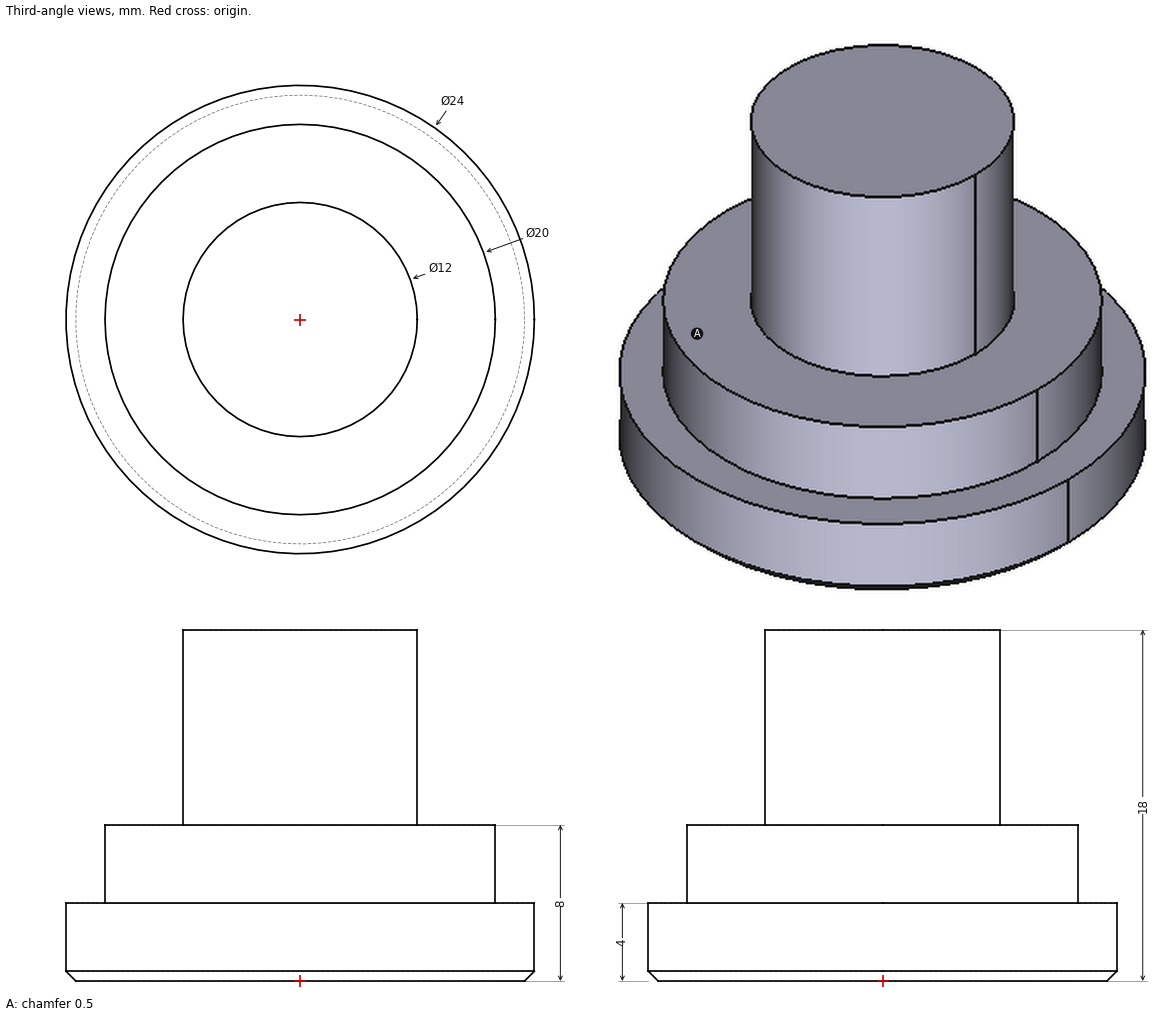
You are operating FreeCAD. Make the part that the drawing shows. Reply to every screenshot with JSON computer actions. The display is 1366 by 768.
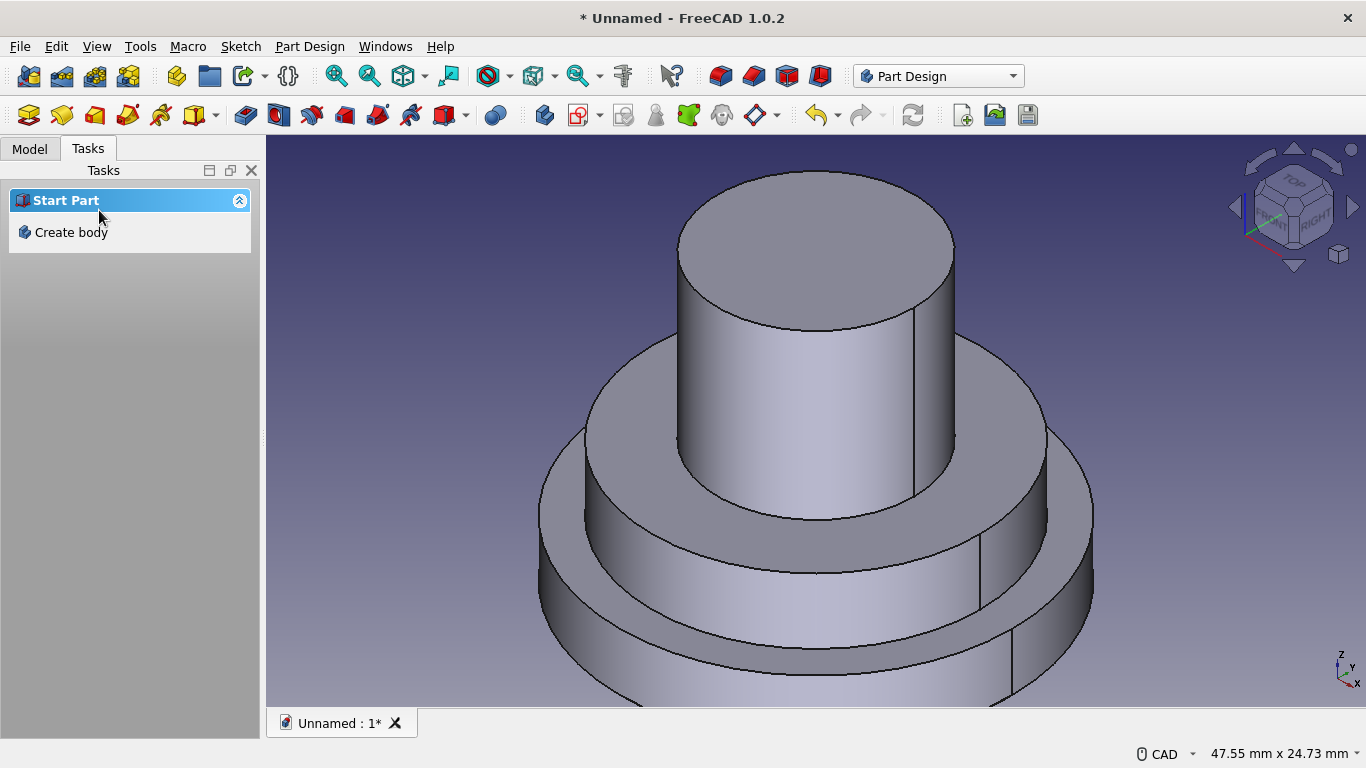
{"action": "left_click", "coordinate": [337, 76]}